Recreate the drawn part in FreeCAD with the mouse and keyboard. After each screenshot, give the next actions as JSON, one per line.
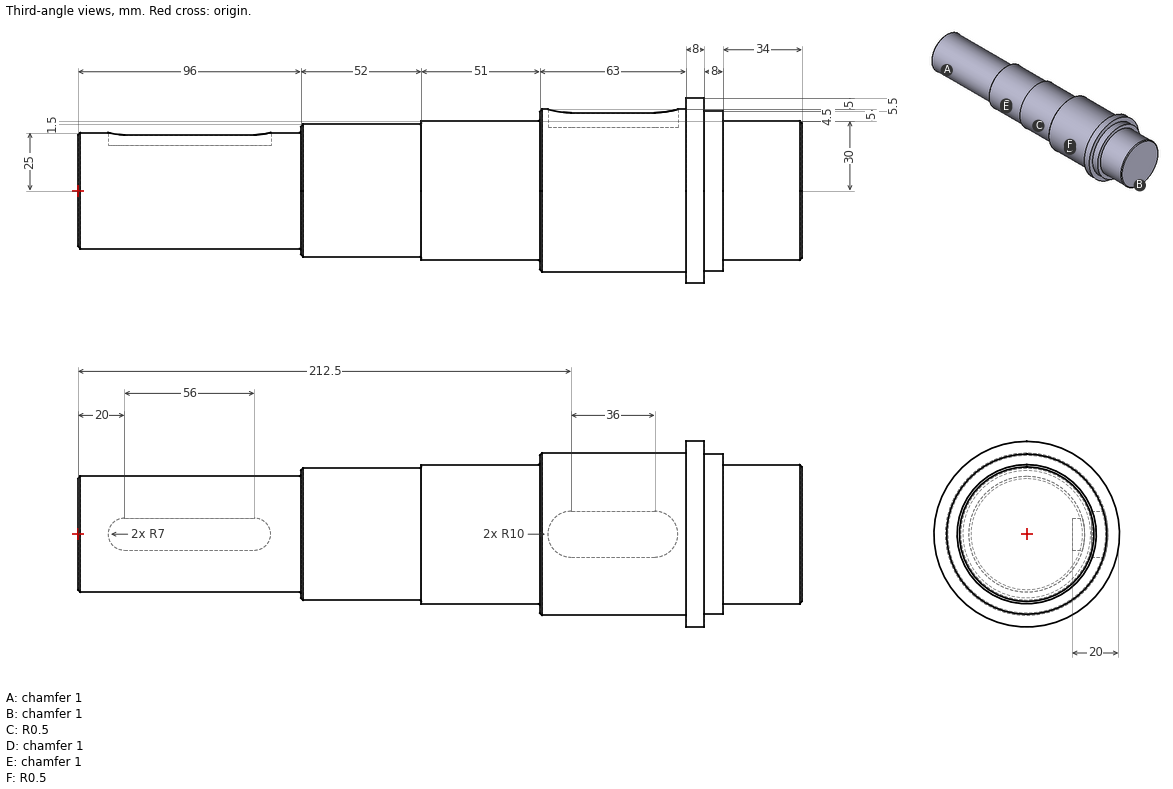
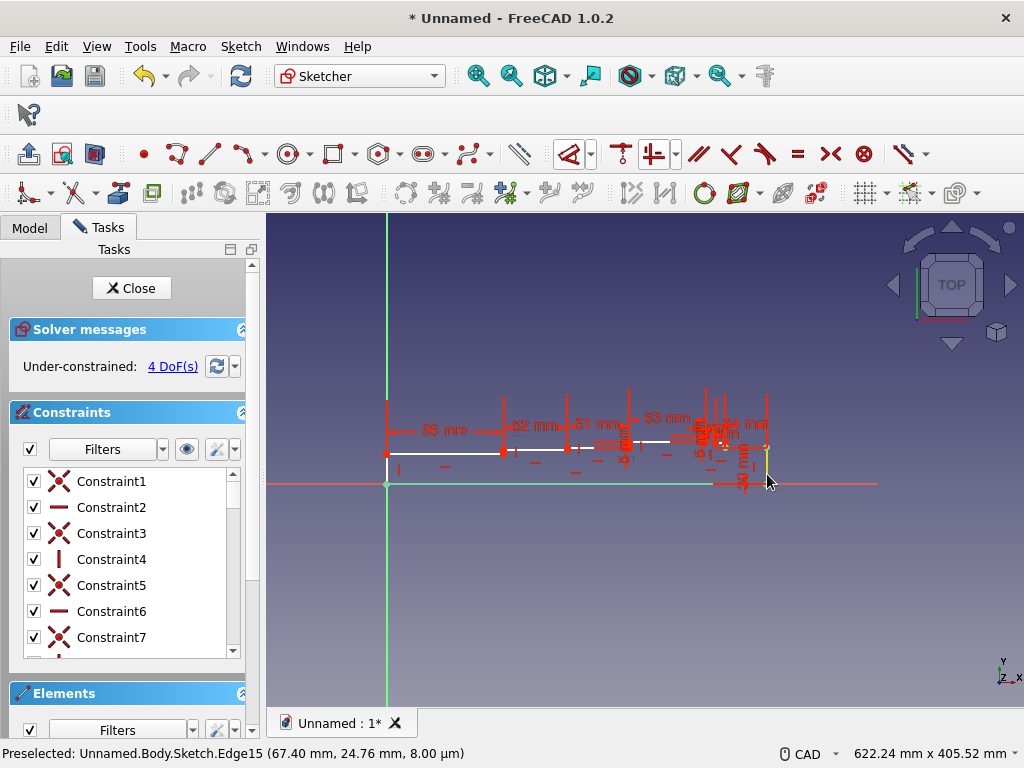
{"action": "scroll", "coordinate": [387, 463], "scroll_direction": "up", "scroll_amount": 3}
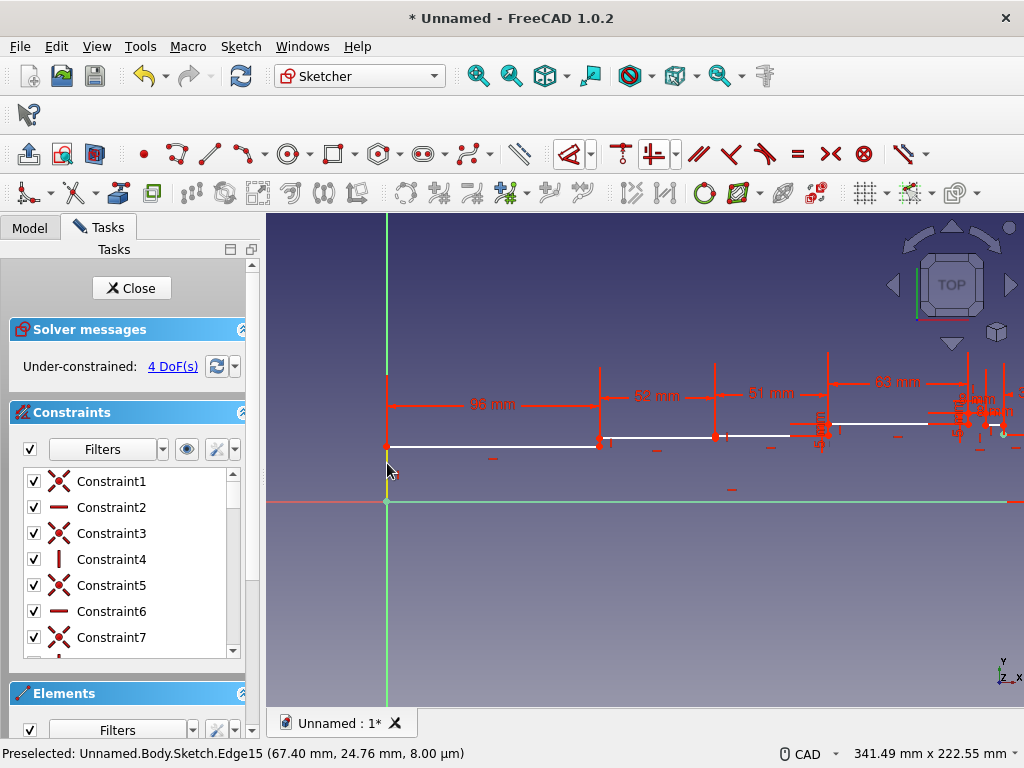
{"action": "left_click", "coordinate": [387, 463]}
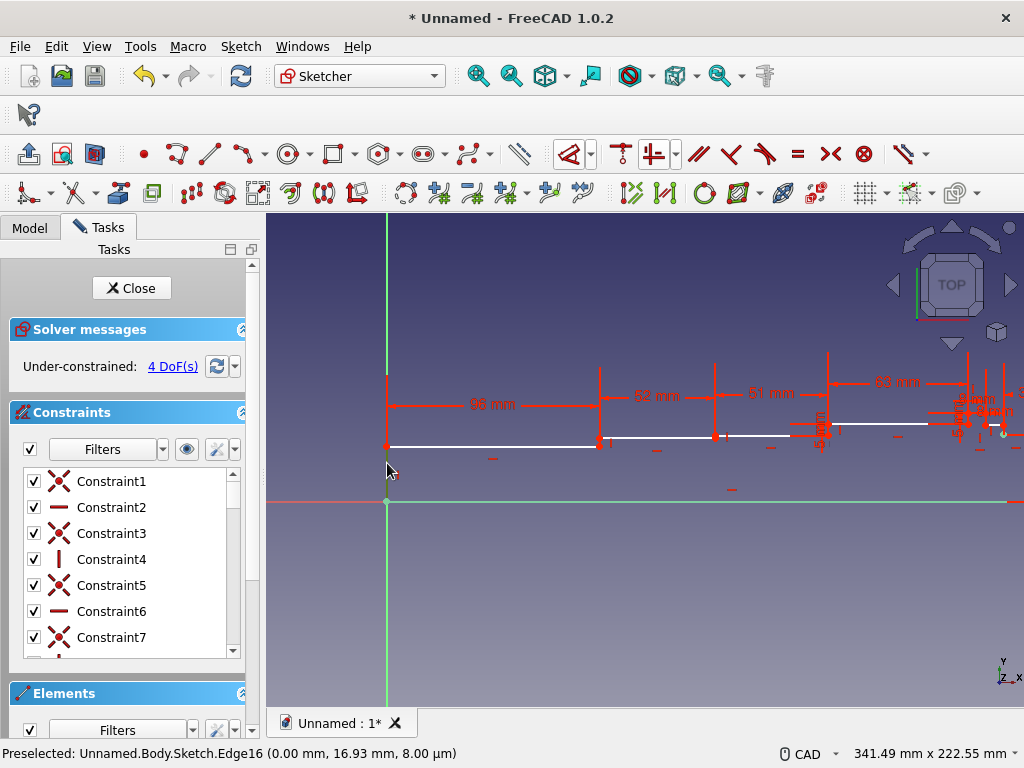
{"action": "key", "text": "i"}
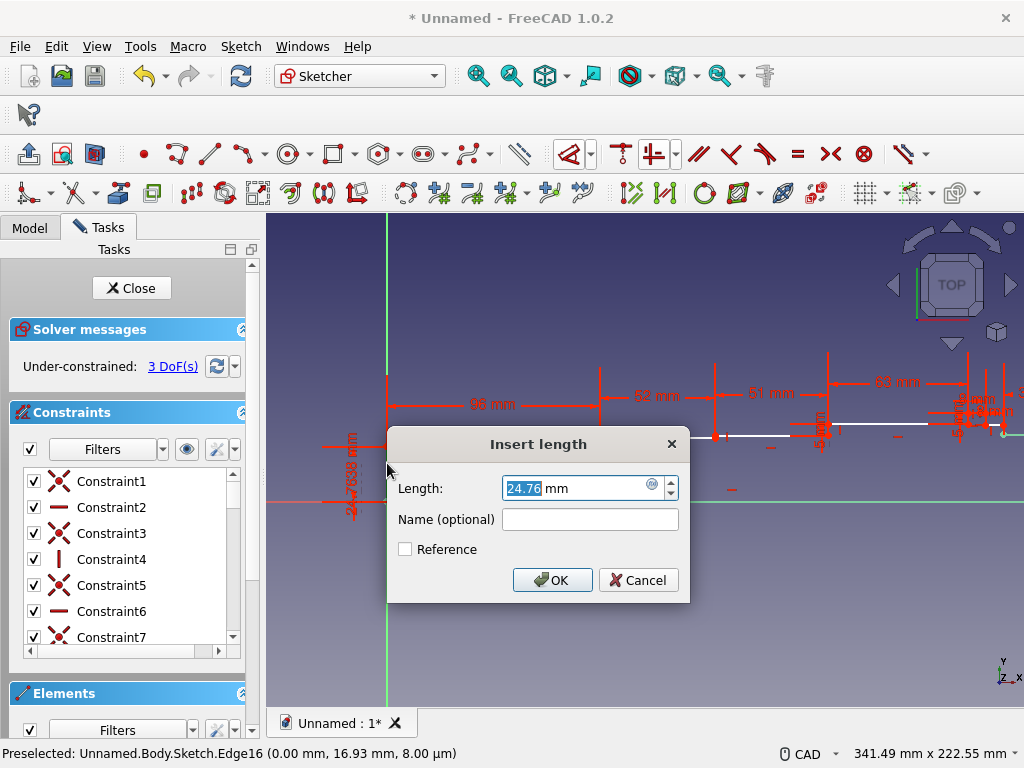
{"action": "type", "text": "25"}
{"action": "key", "text": "Return"}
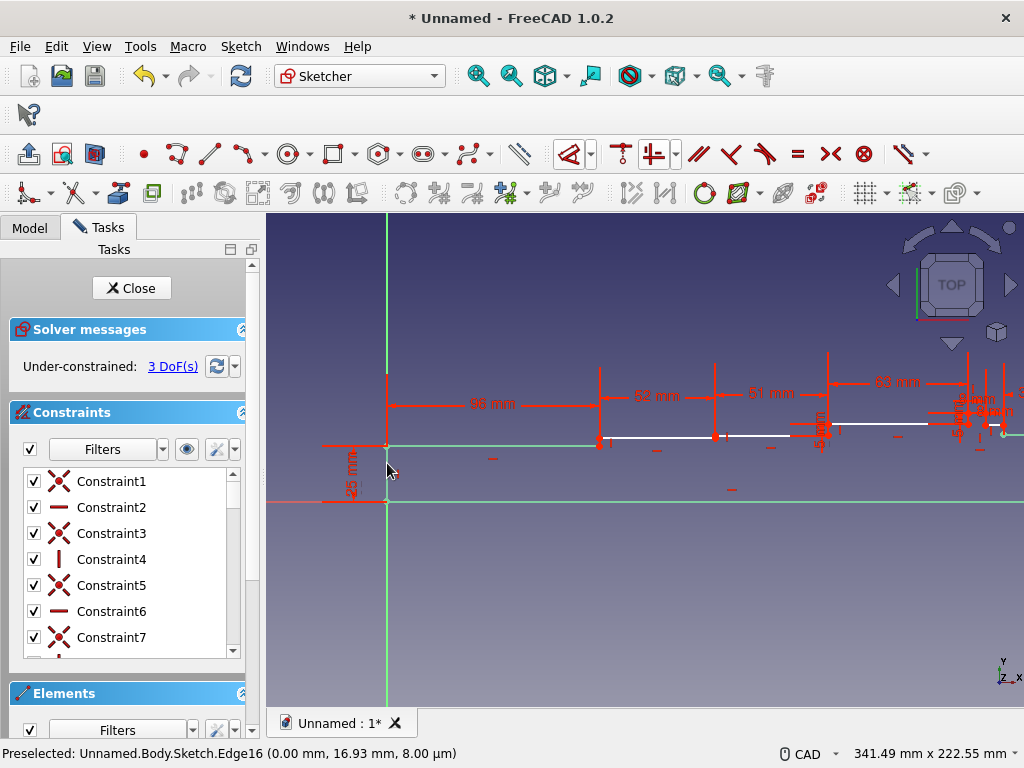
{"action": "scroll", "coordinate": [386, 463], "scroll_direction": "down", "scroll_amount": 3}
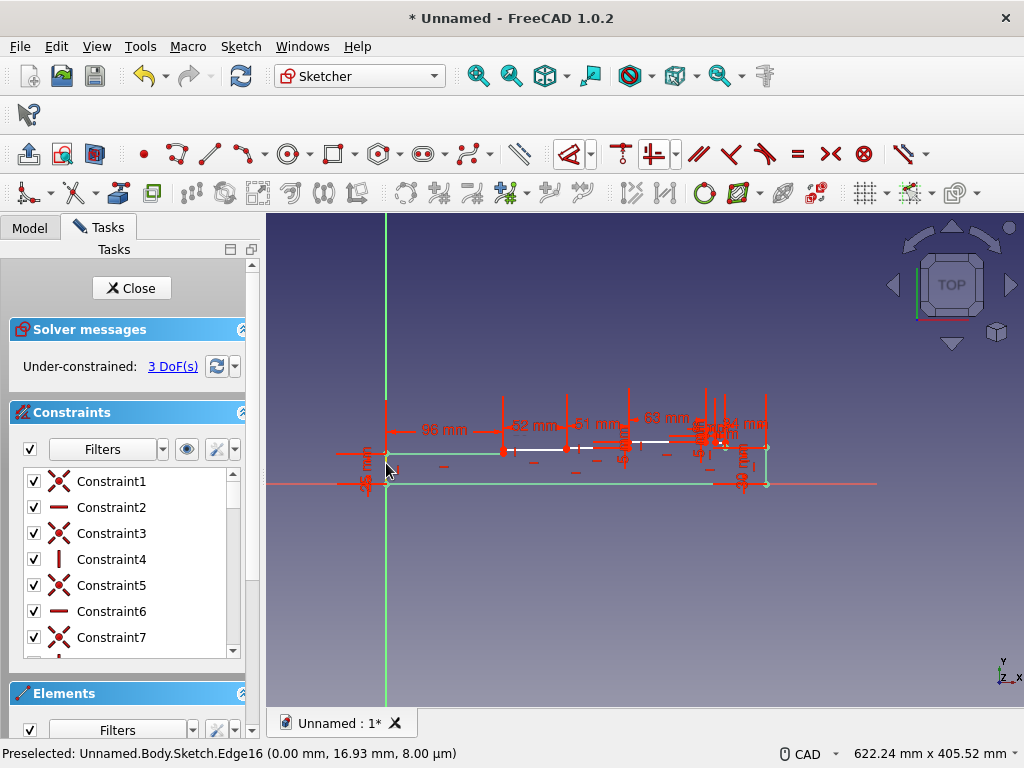
{"action": "scroll", "coordinate": [725, 445], "scroll_direction": "up", "scroll_amount": 10}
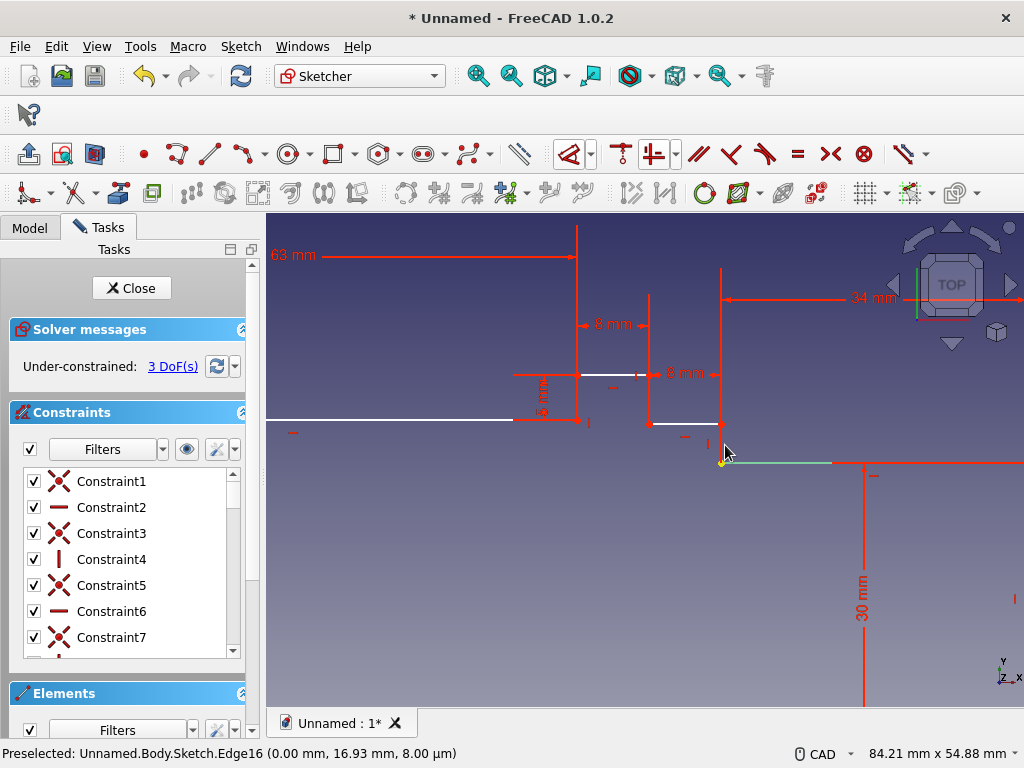
{"action": "left_click", "coordinate": [721, 444]}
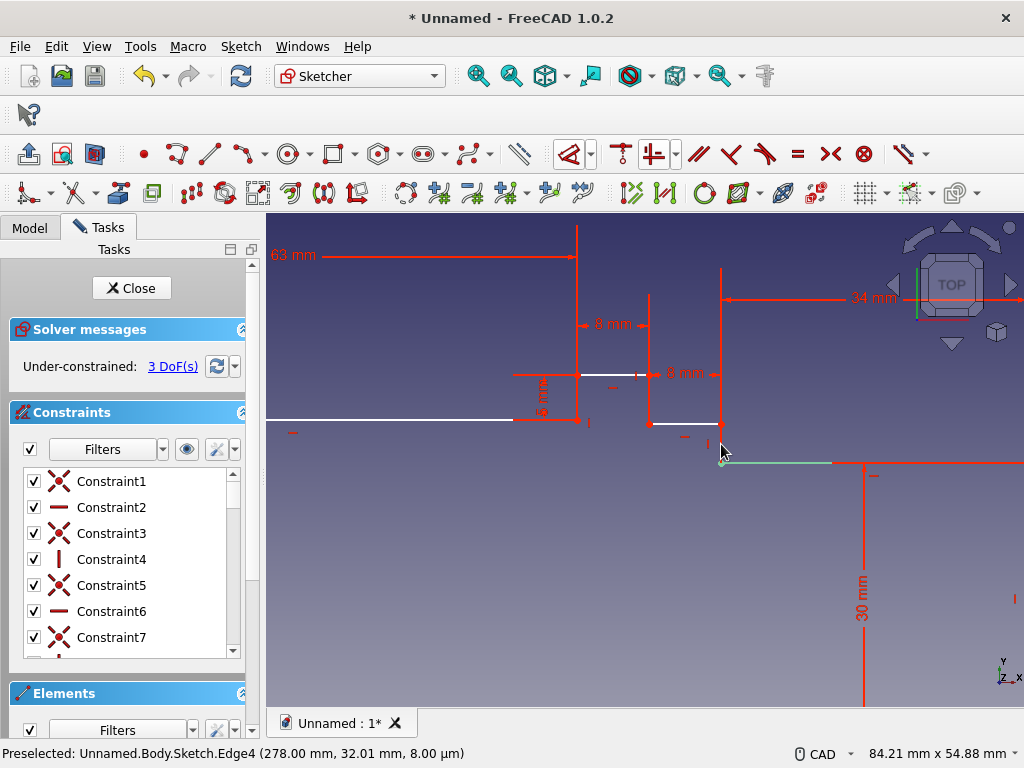
{"action": "key", "text": "i"}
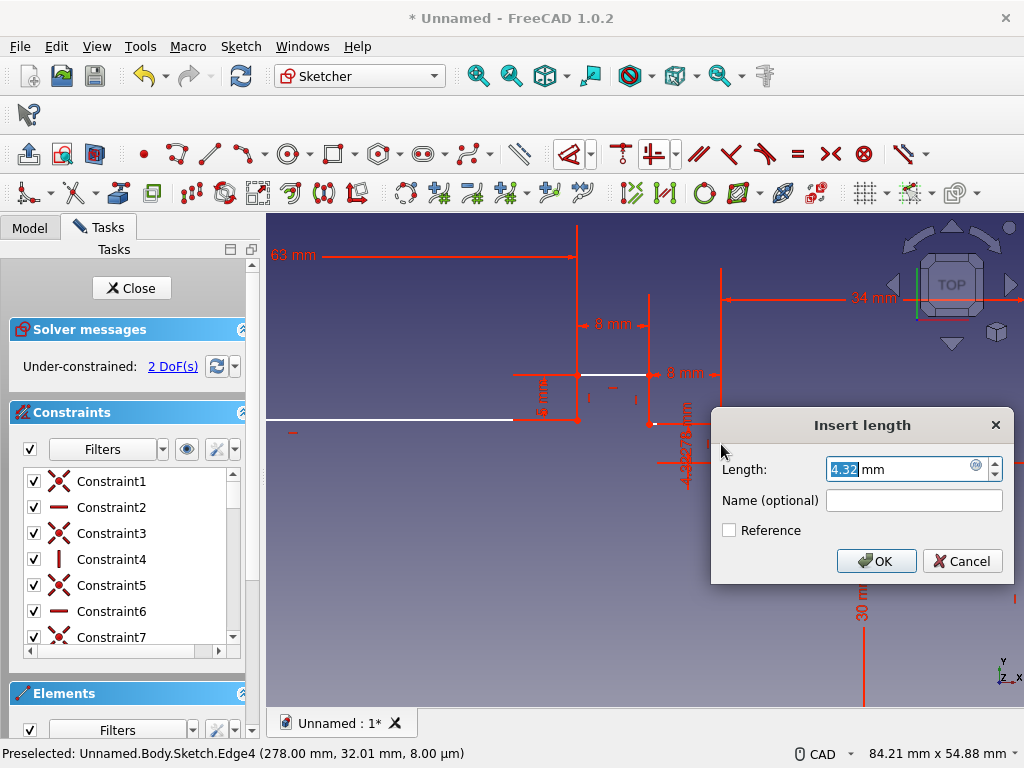
{"action": "type", "text": "4.5"}
{"action": "key", "text": "Return"}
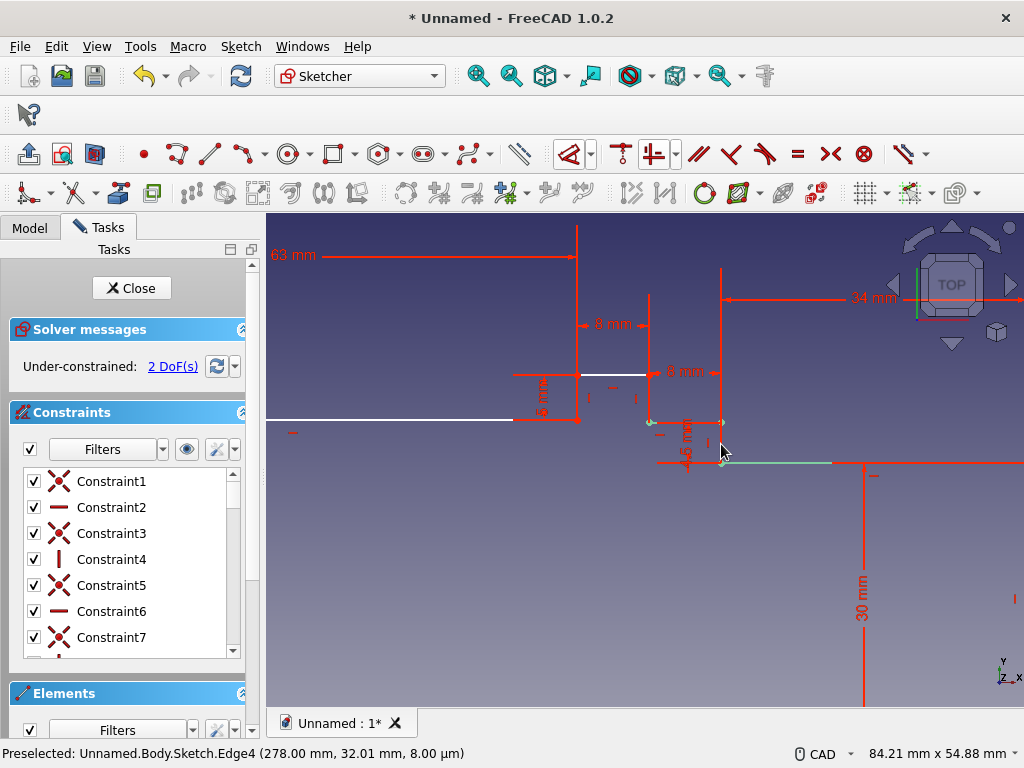
{"action": "left_click", "coordinate": [649, 408]}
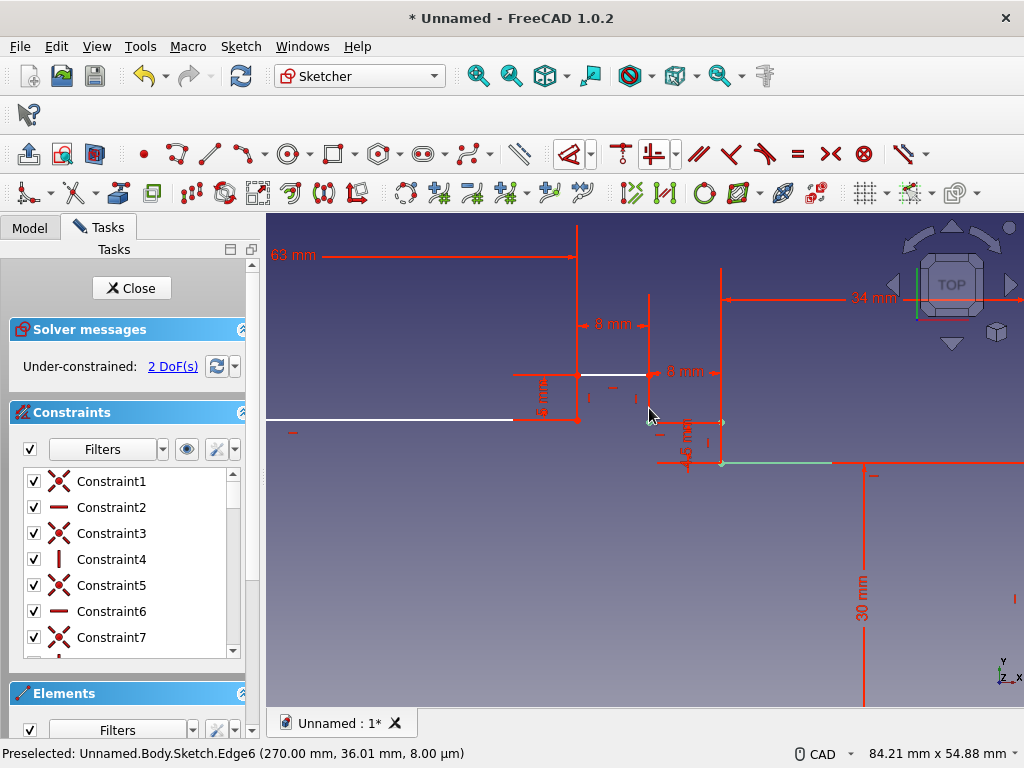
{"action": "key", "text": "i"}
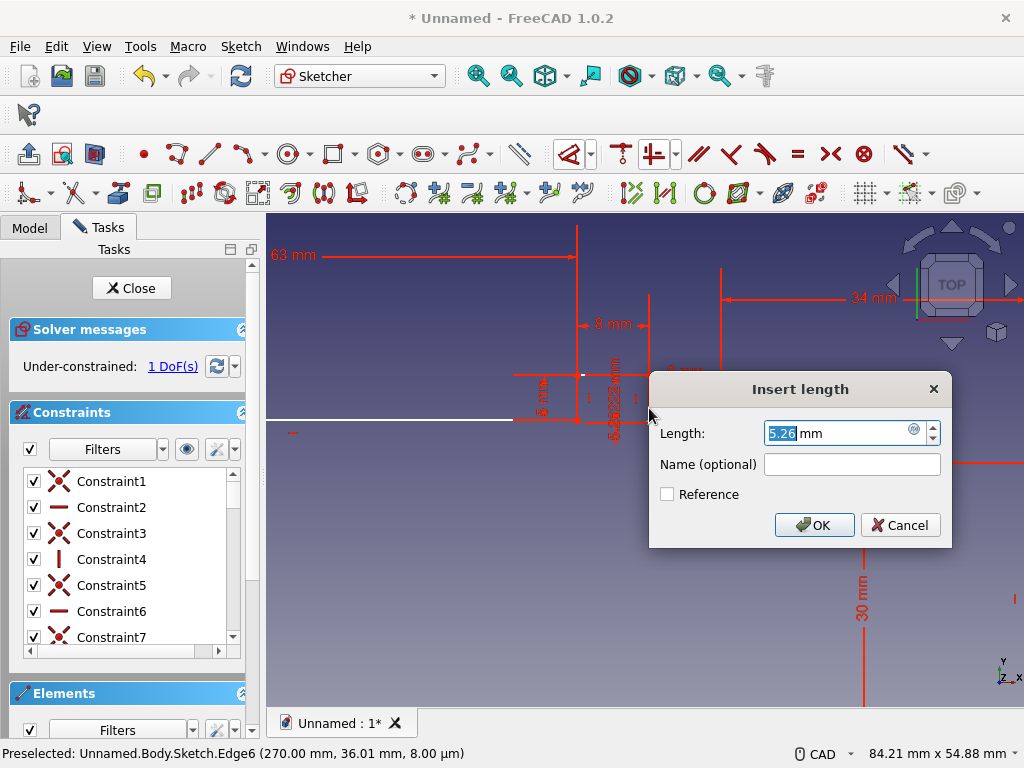
{"action": "type", "text": "5.5"}
{"action": "key", "text": "Return"}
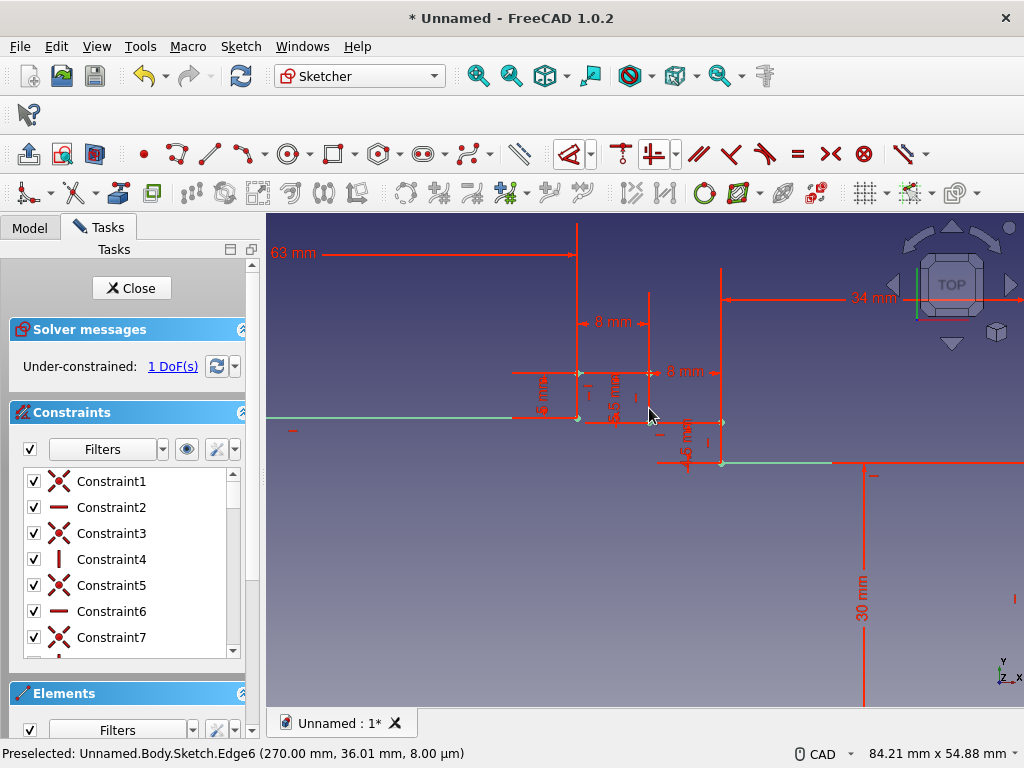
{"action": "scroll", "coordinate": [726, 445], "scroll_direction": "down", "scroll_amount": 10}